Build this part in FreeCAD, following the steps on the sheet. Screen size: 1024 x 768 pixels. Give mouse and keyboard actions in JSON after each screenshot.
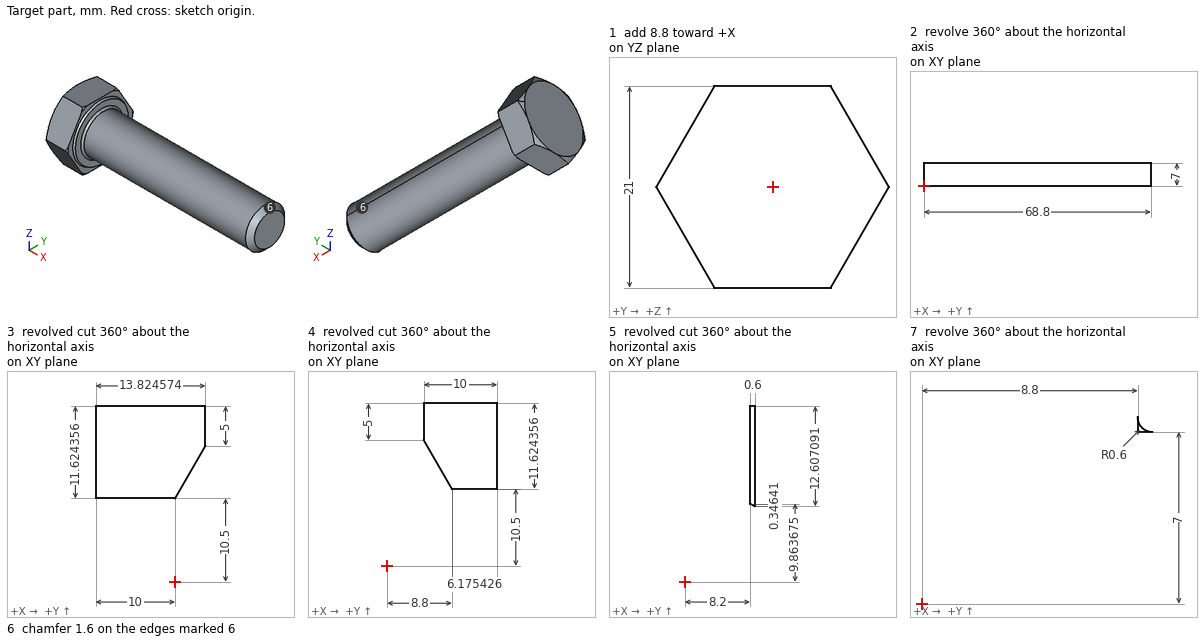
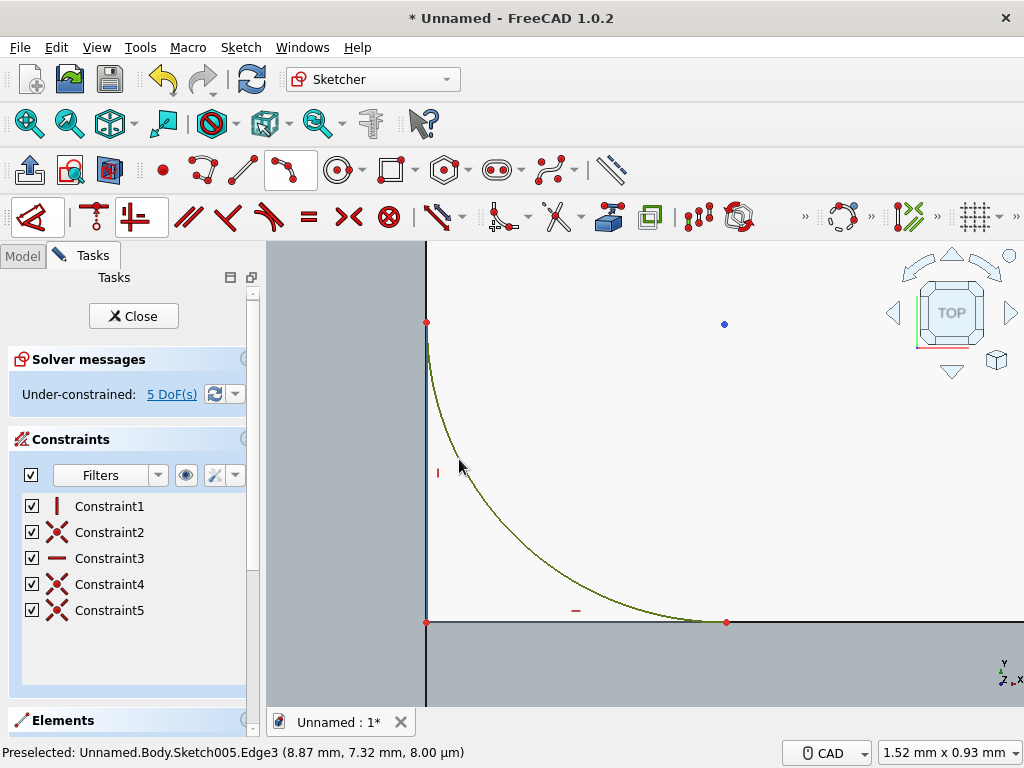
{"action": "left_click", "coordinate": [270, 218]}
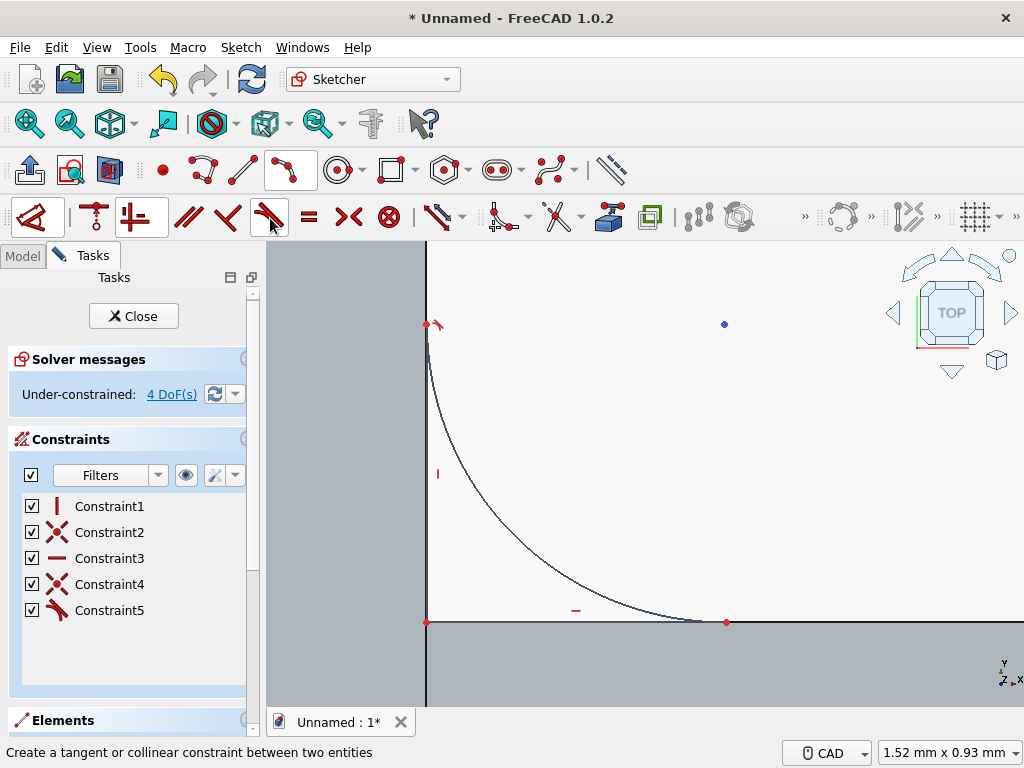
{"action": "left_click", "coordinate": [517, 622]}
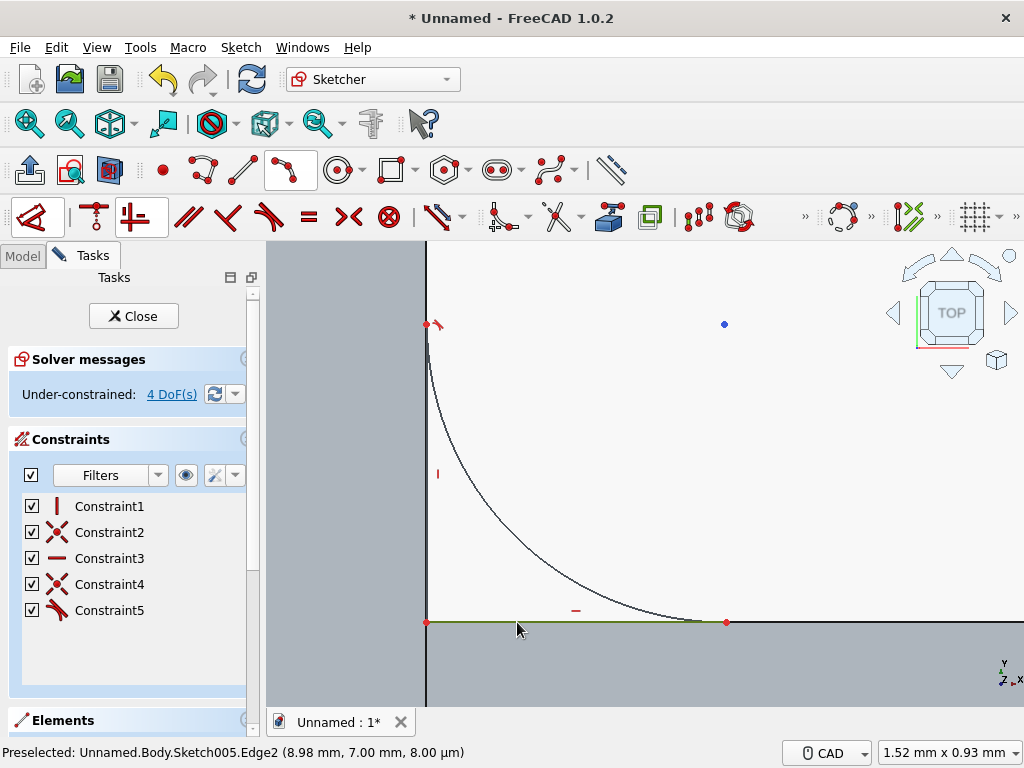
{"action": "left_click", "coordinate": [460, 460]}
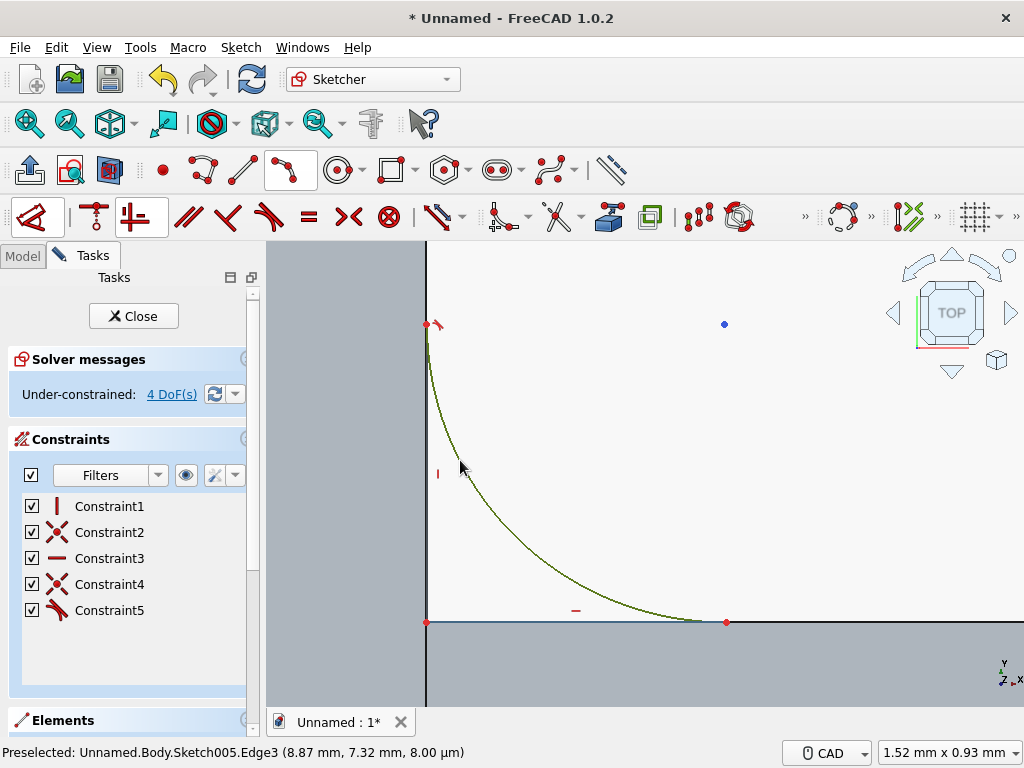
{"action": "left_click", "coordinate": [270, 218]}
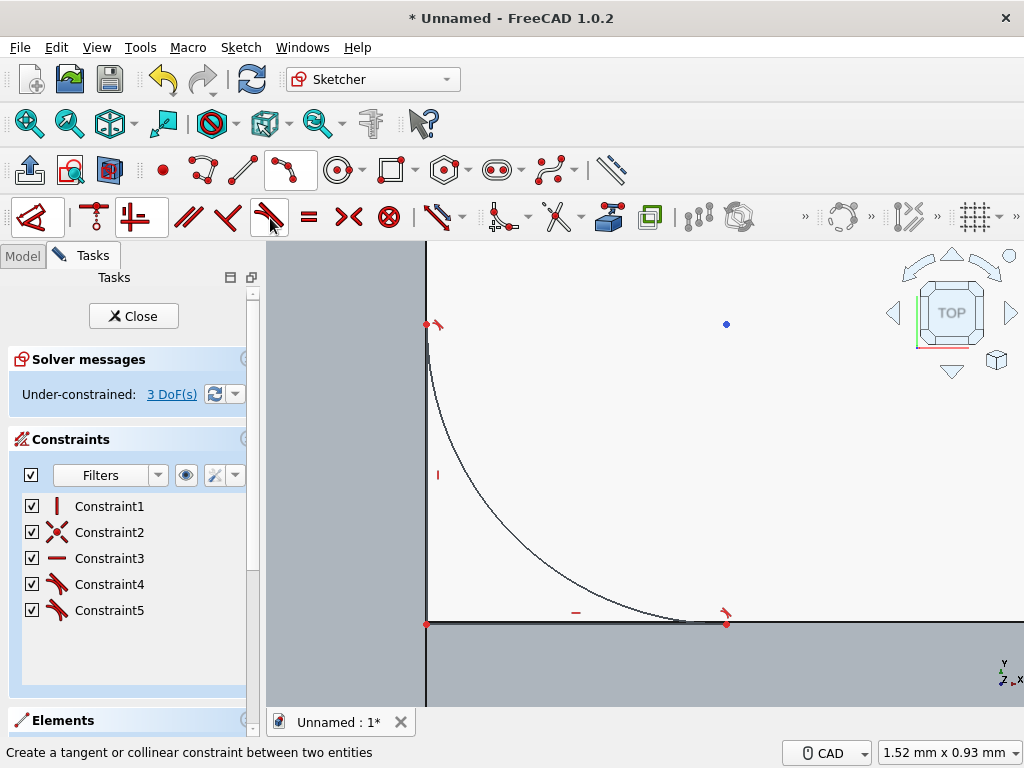
{"action": "left_click", "coordinate": [460, 461]}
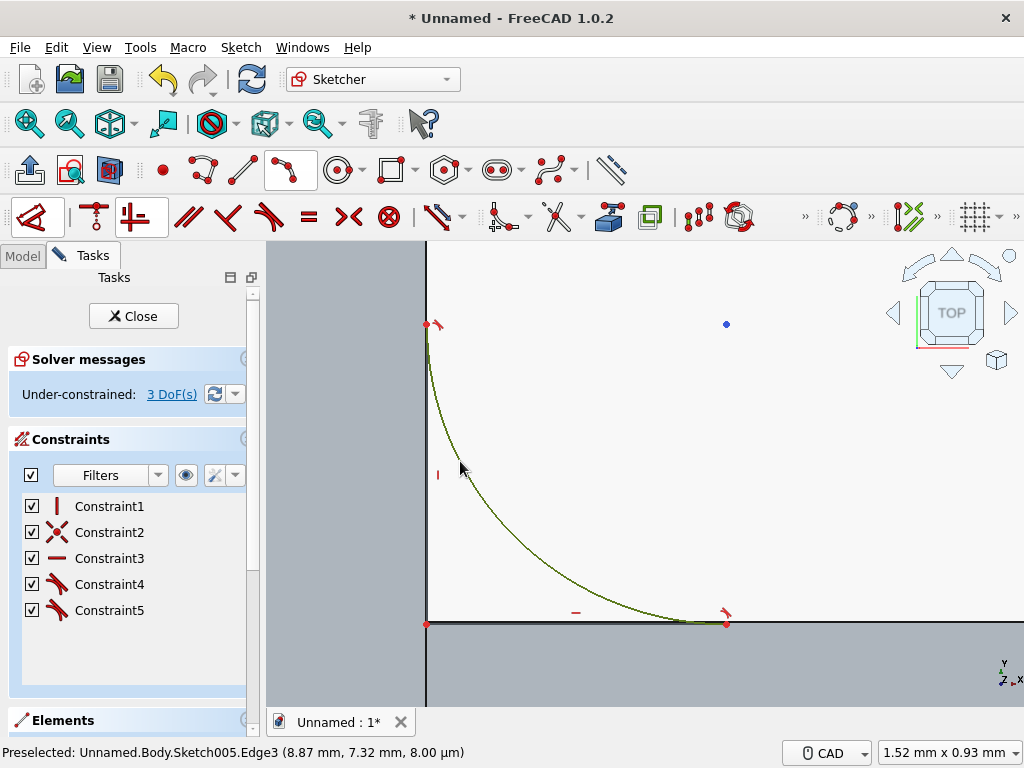
{"action": "left_click", "coordinate": [58, 218]}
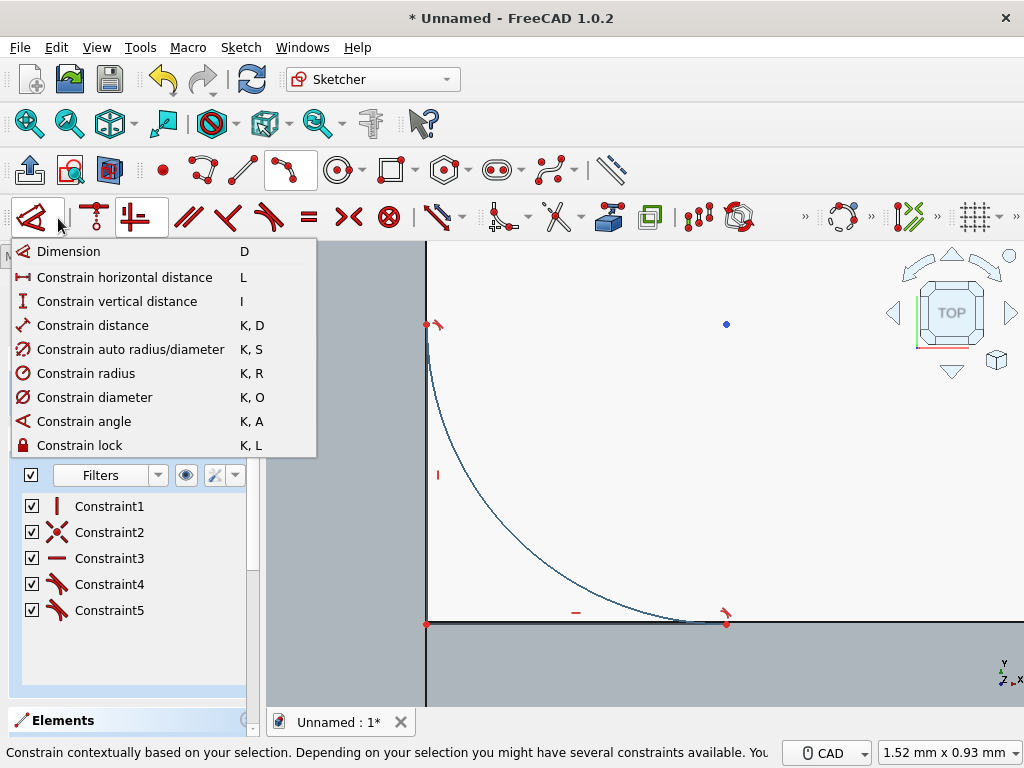
{"action": "left_click", "coordinate": [164, 373]}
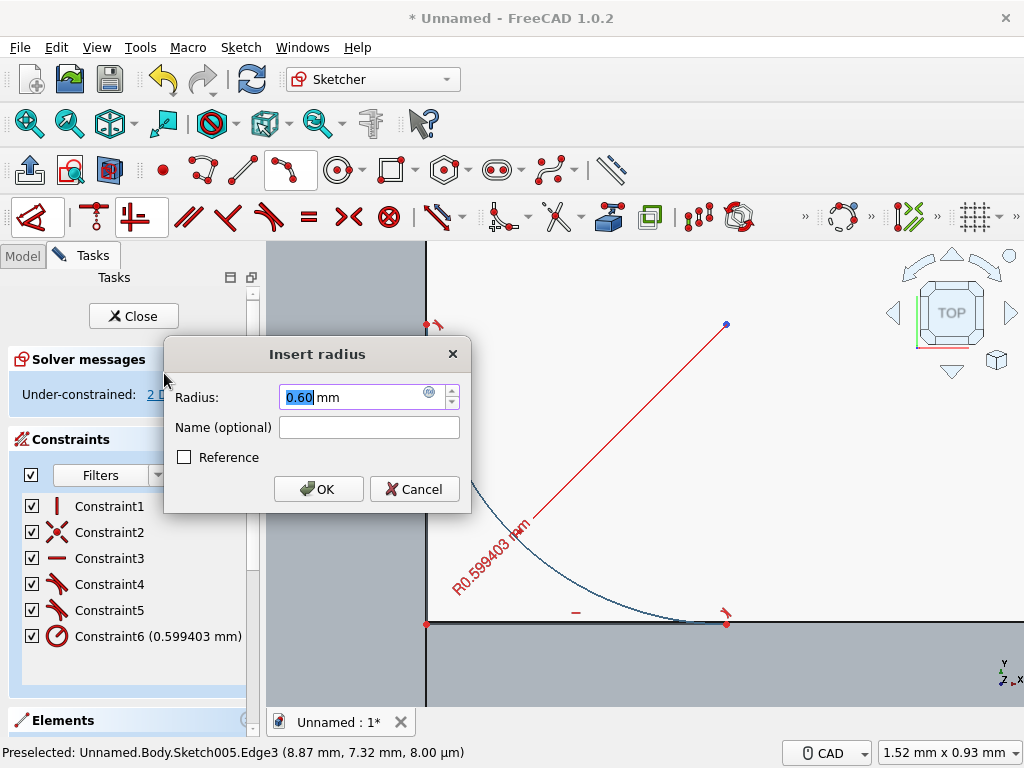
{"action": "type", "text": "0.6"}
{"action": "key", "text": "Return"}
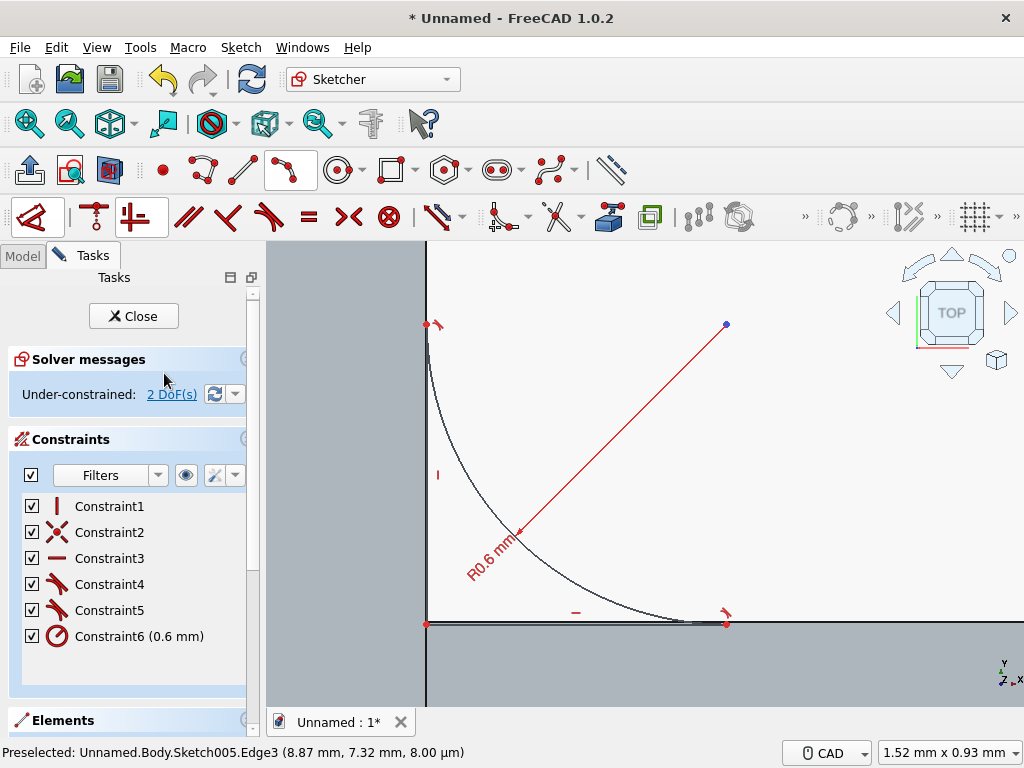
{"action": "left_click", "coordinate": [427, 625]}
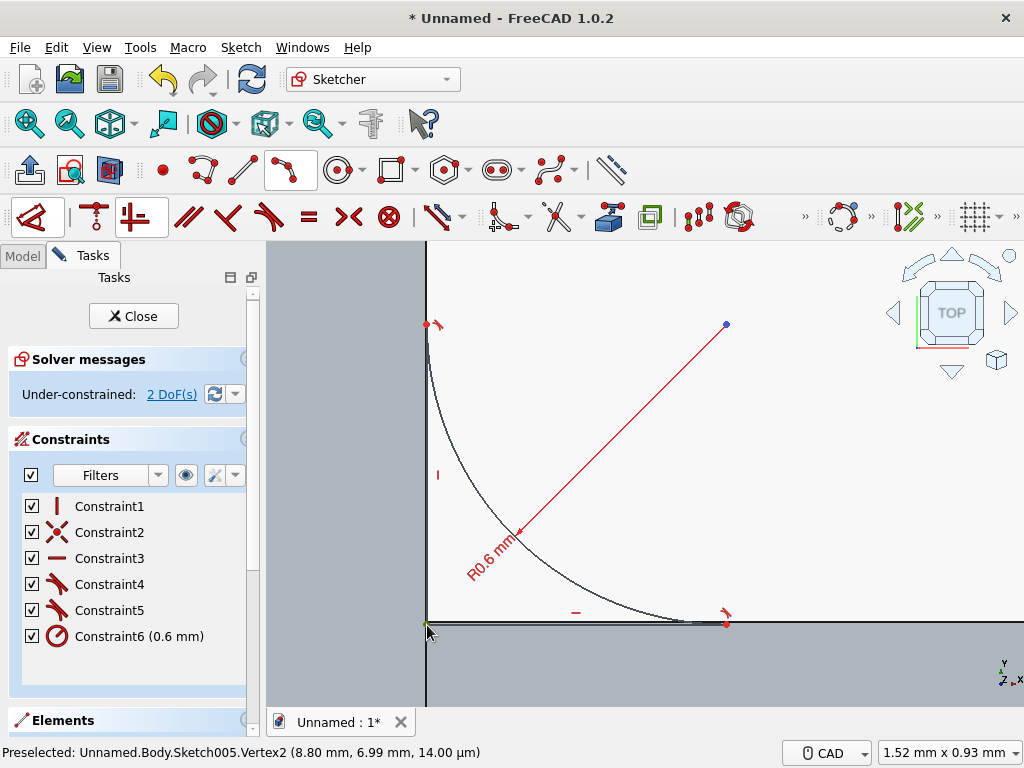
{"action": "left_click", "coordinate": [58, 218]}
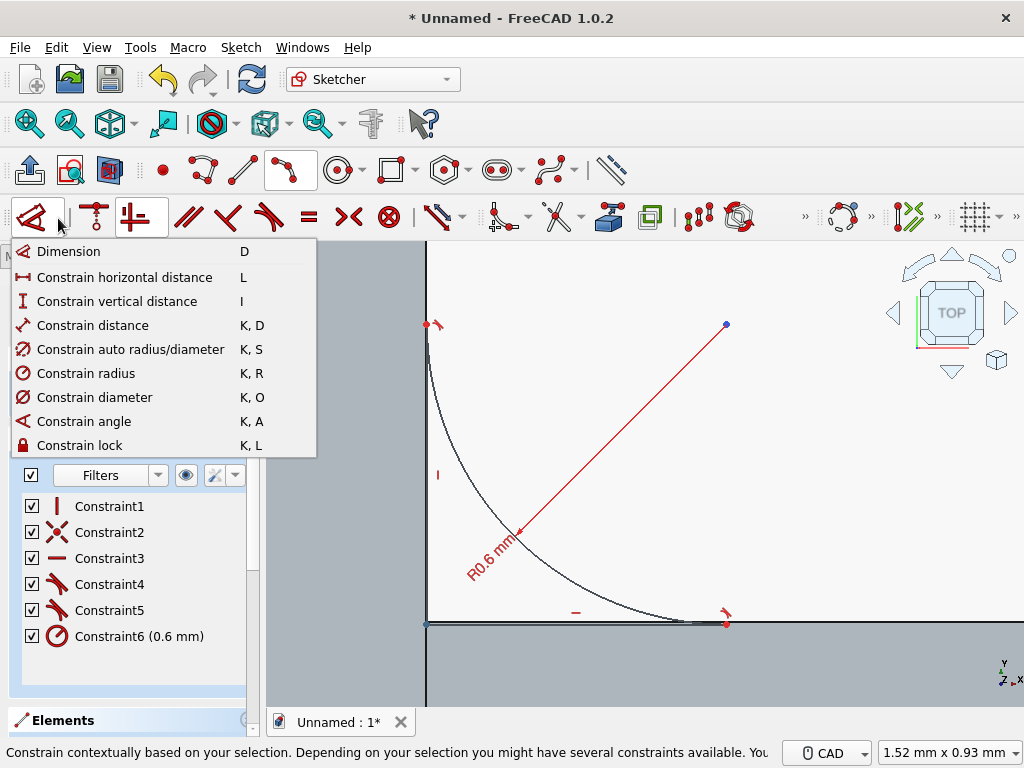
{"action": "left_click", "coordinate": [164, 301]}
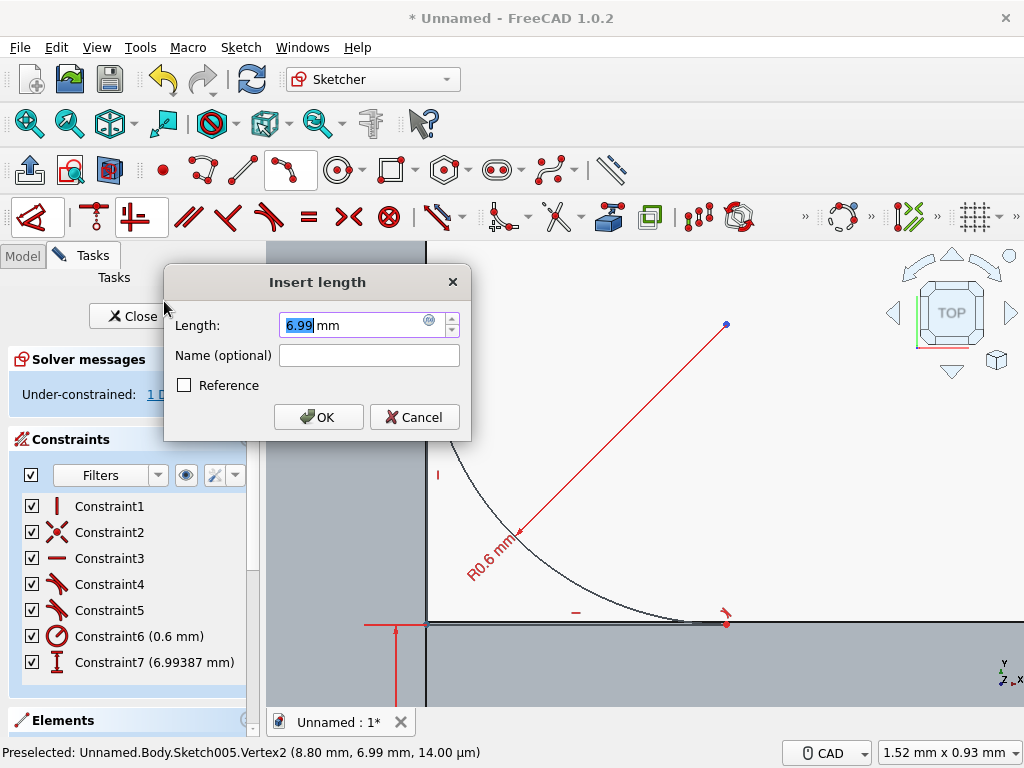
{"action": "type", "text": "7"}
{"action": "key", "text": "Return"}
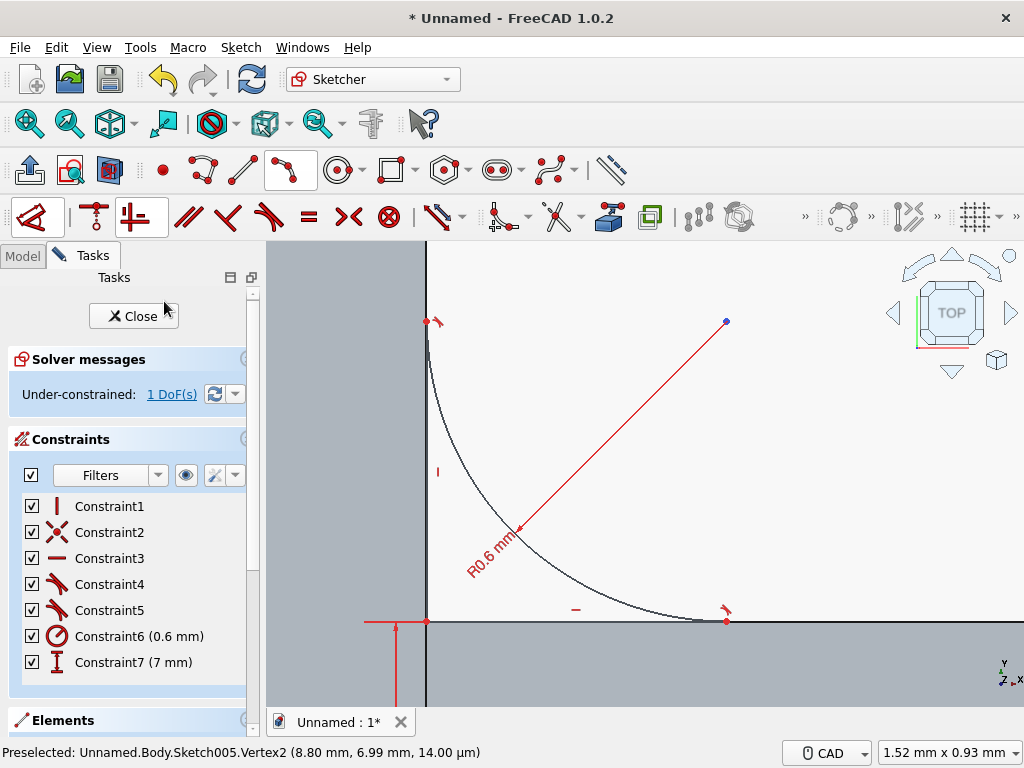
{"action": "left_click", "coordinate": [427, 322]}